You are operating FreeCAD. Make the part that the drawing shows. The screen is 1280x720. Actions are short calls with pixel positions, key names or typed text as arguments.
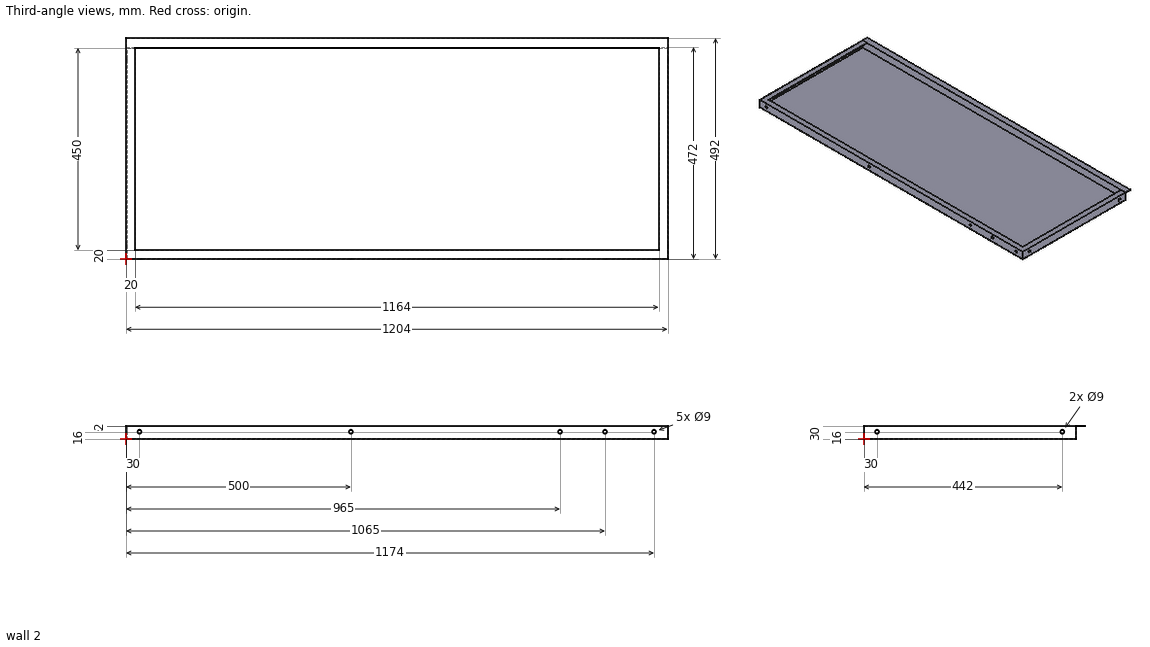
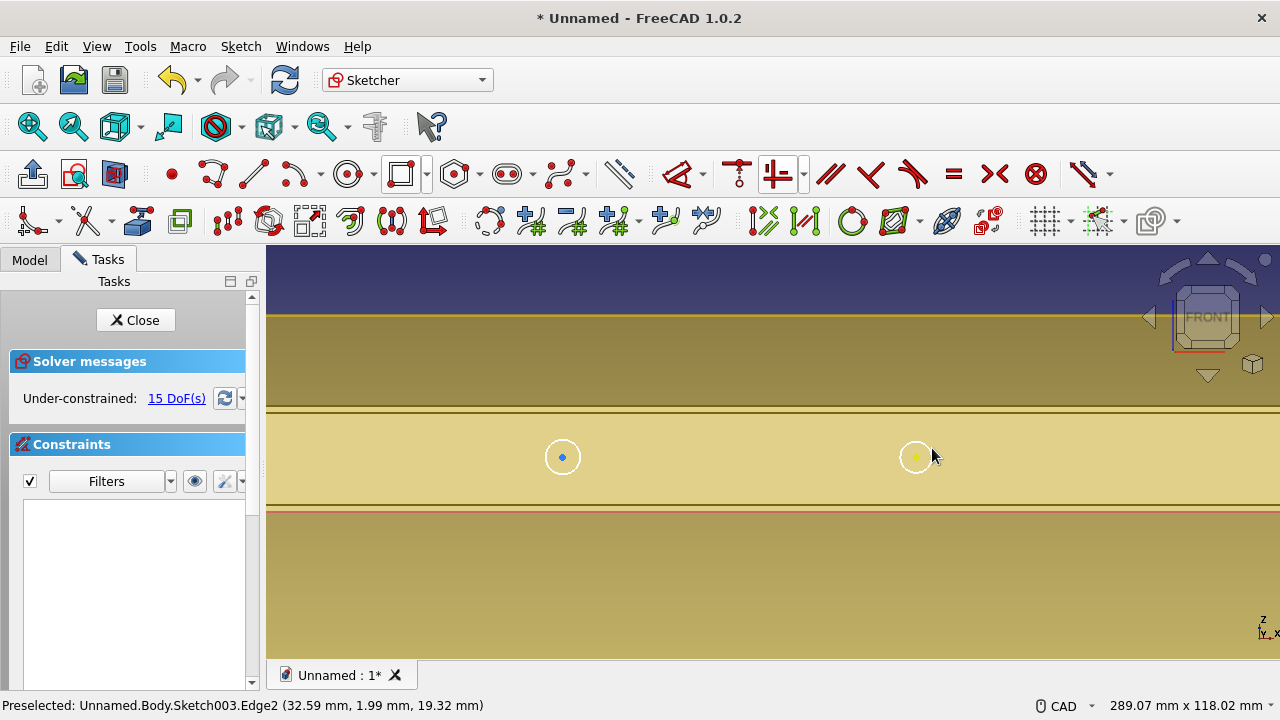
click(927, 446)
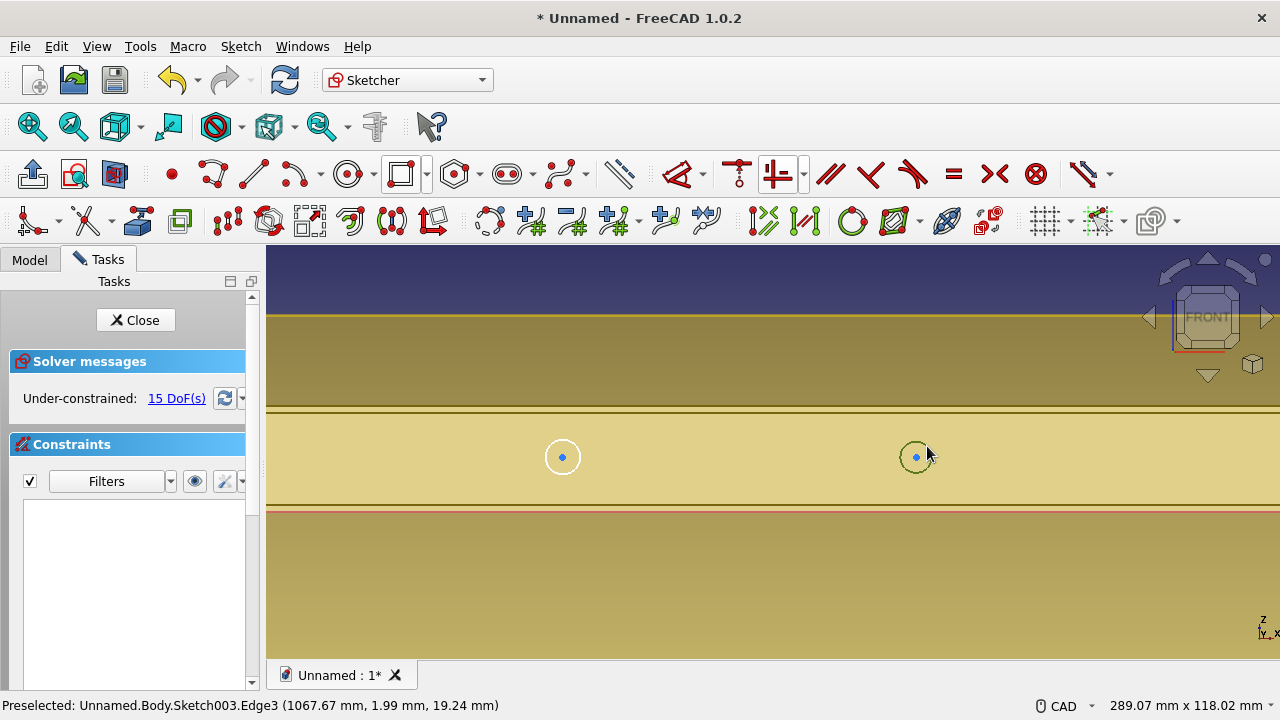
click(575, 445)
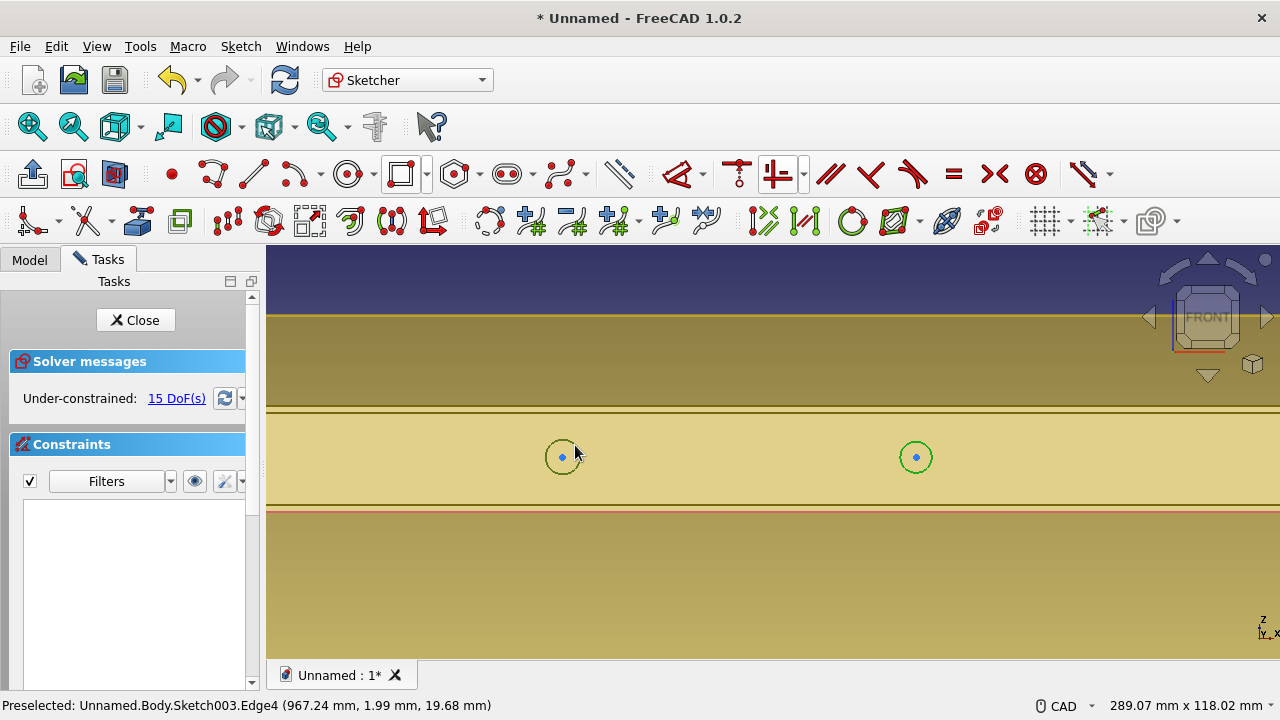
scroll(933, 448, down, 10)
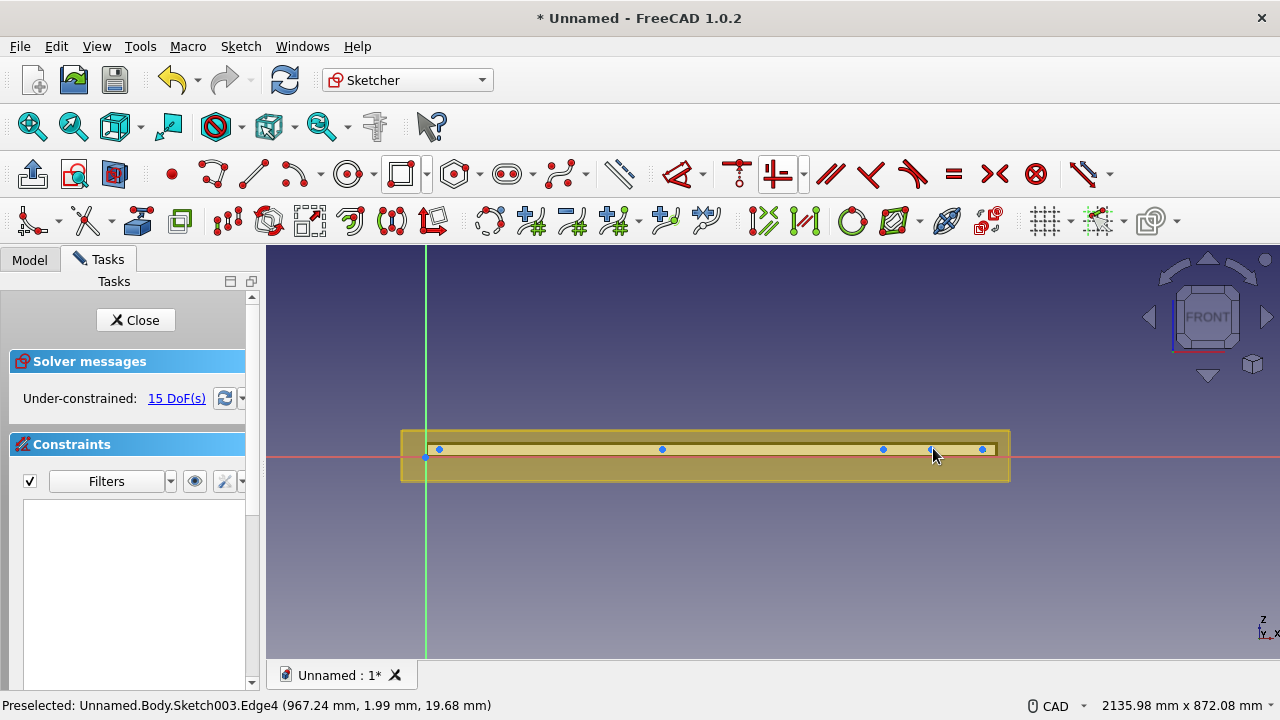
scroll(665, 448, up, 9)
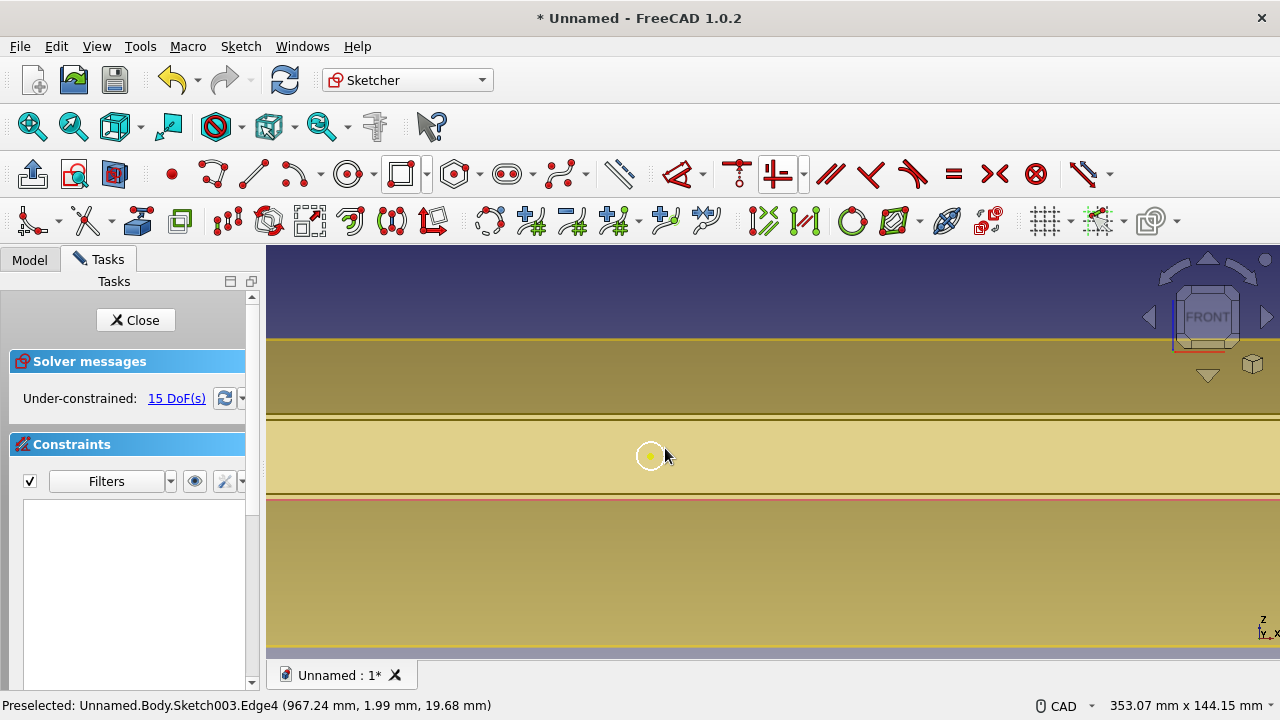
click(660, 446)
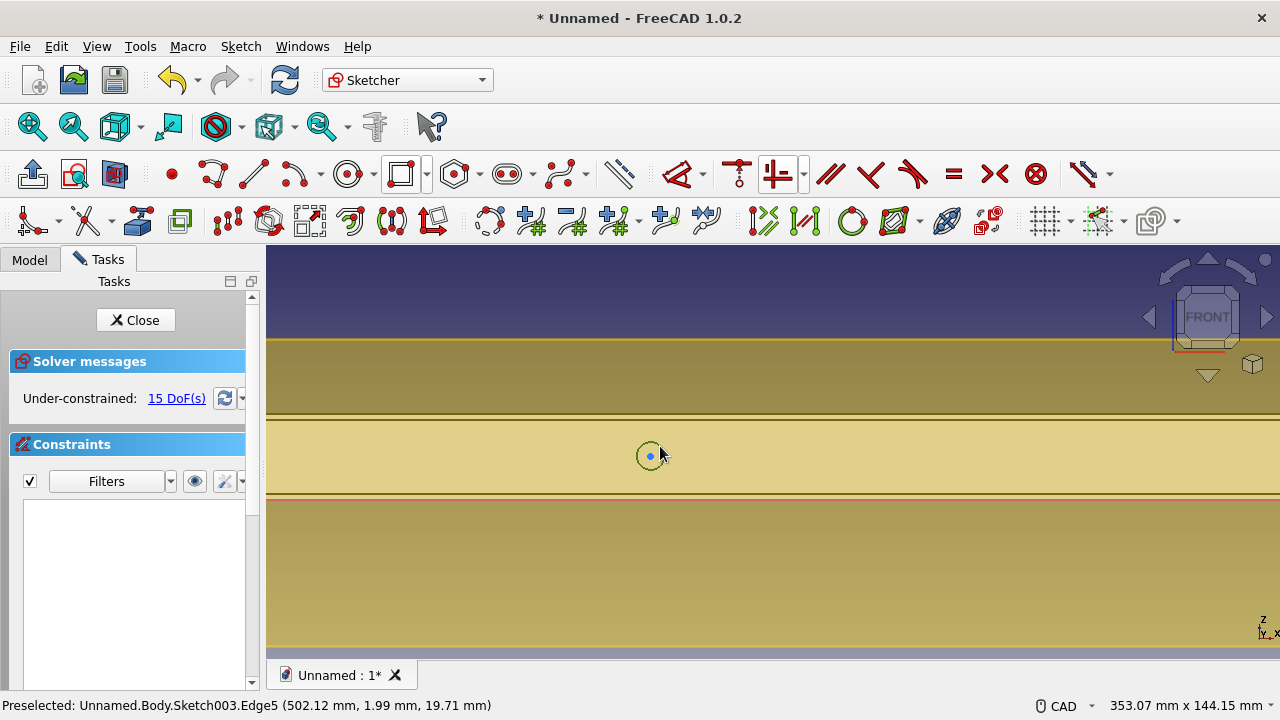
click(954, 174)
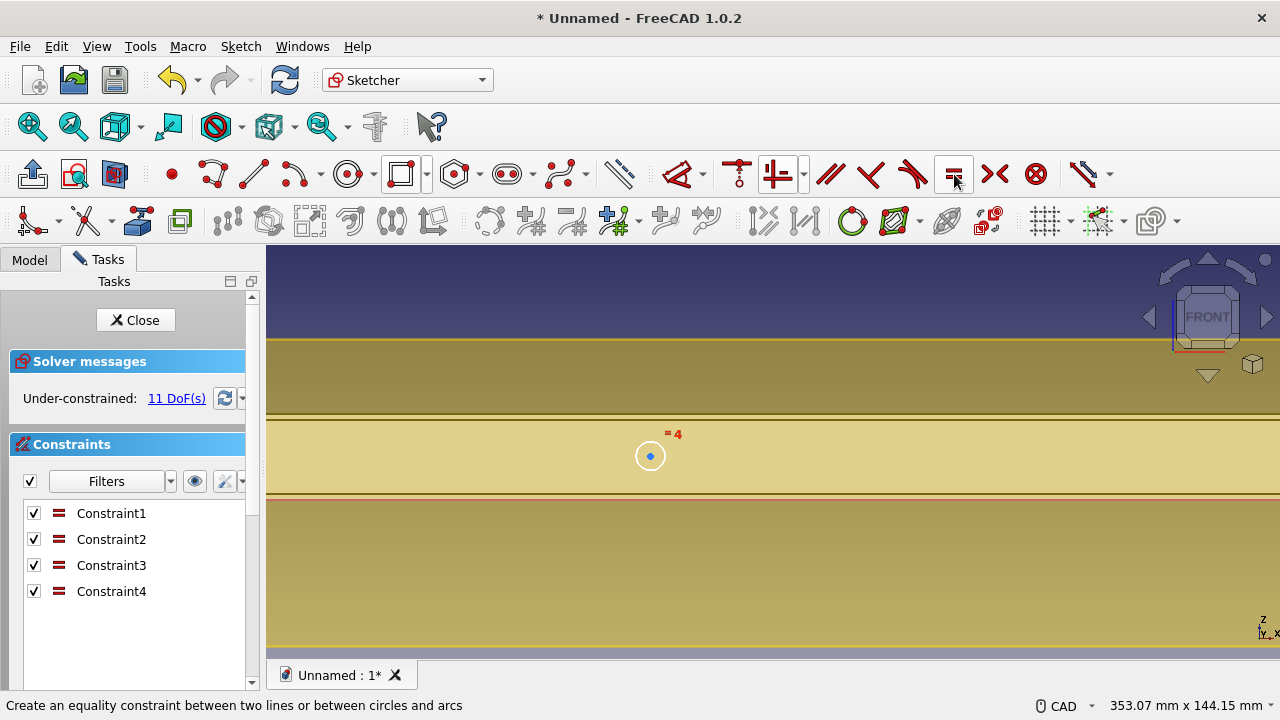
click(676, 174)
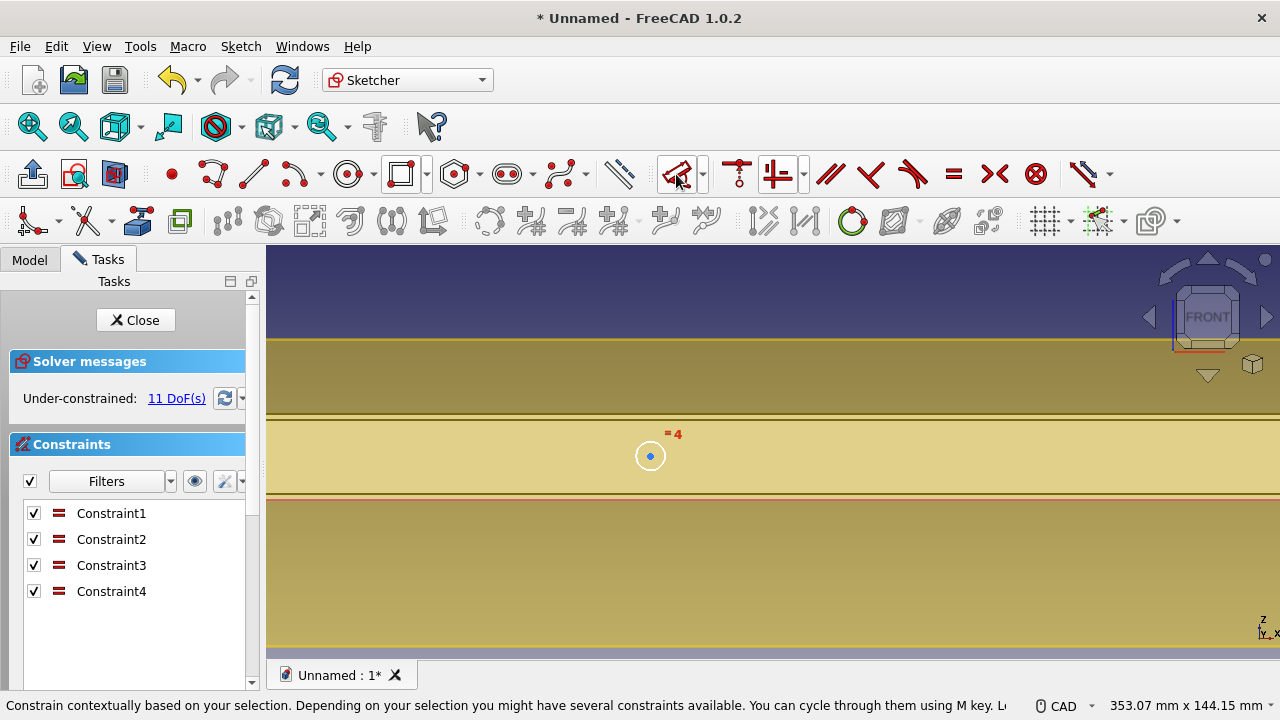
scroll(664, 448, down, 9)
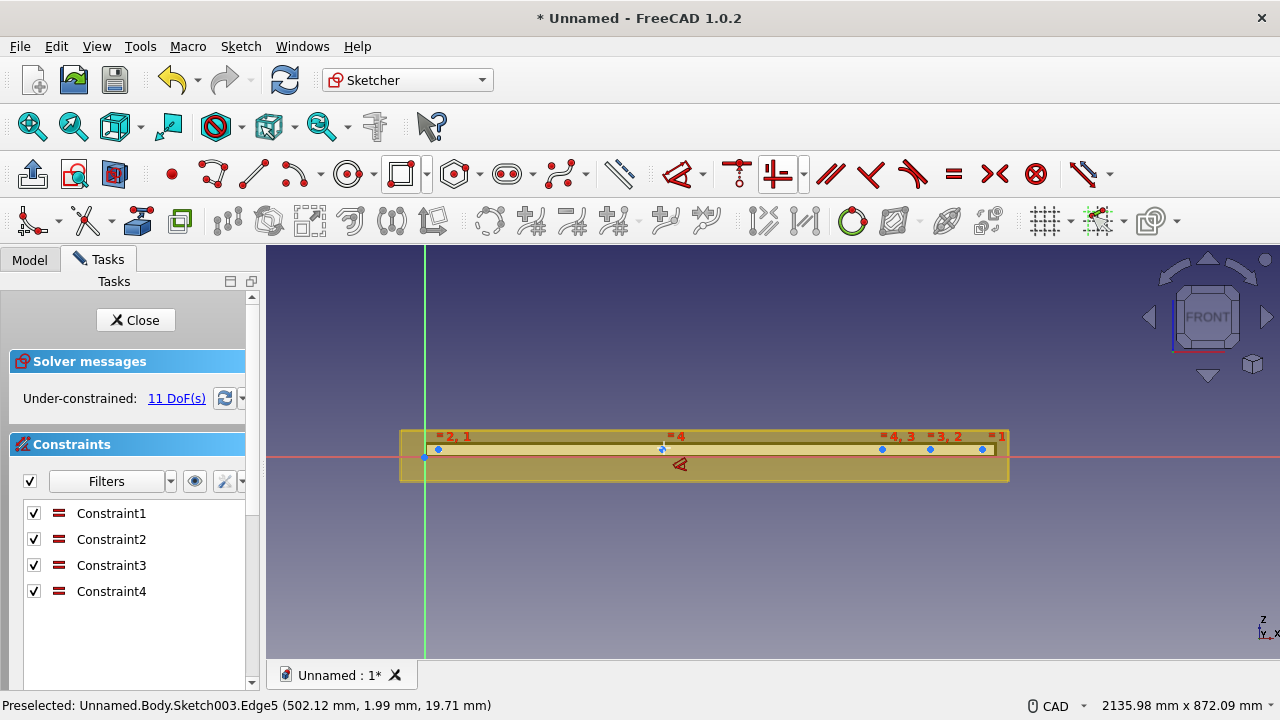
scroll(984, 448, up, 12)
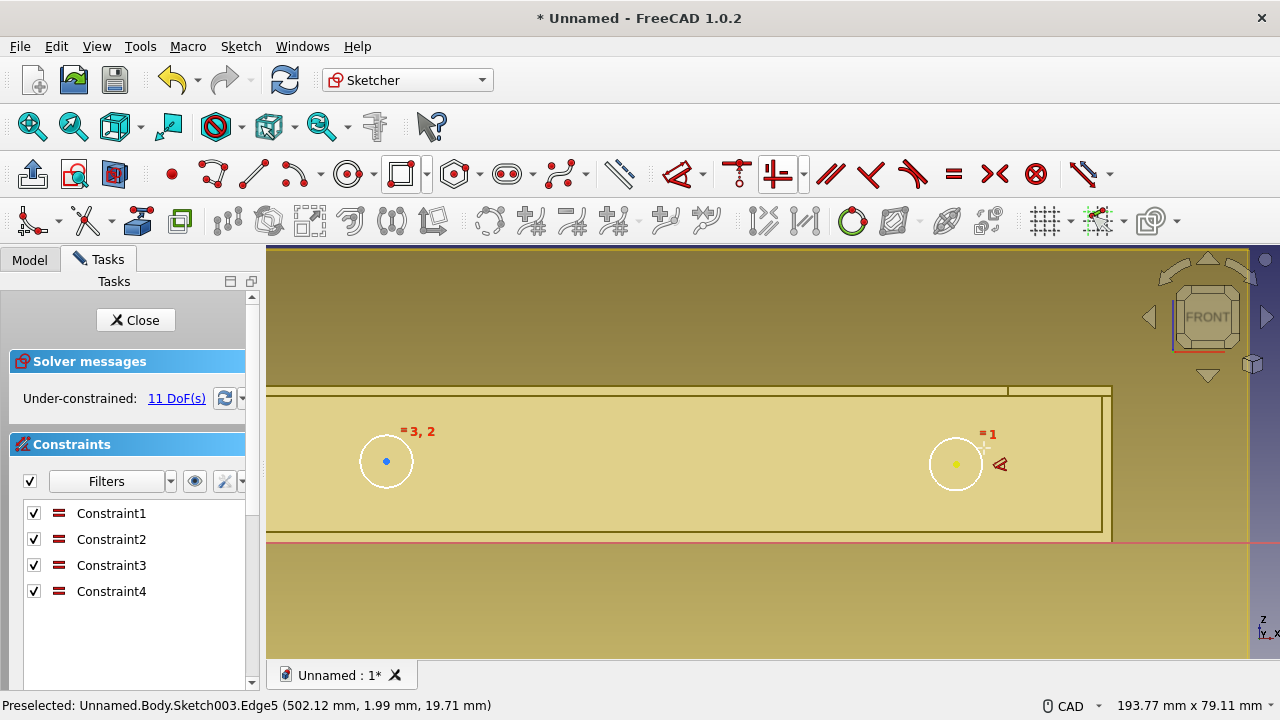
click(974, 446)
click(996, 423)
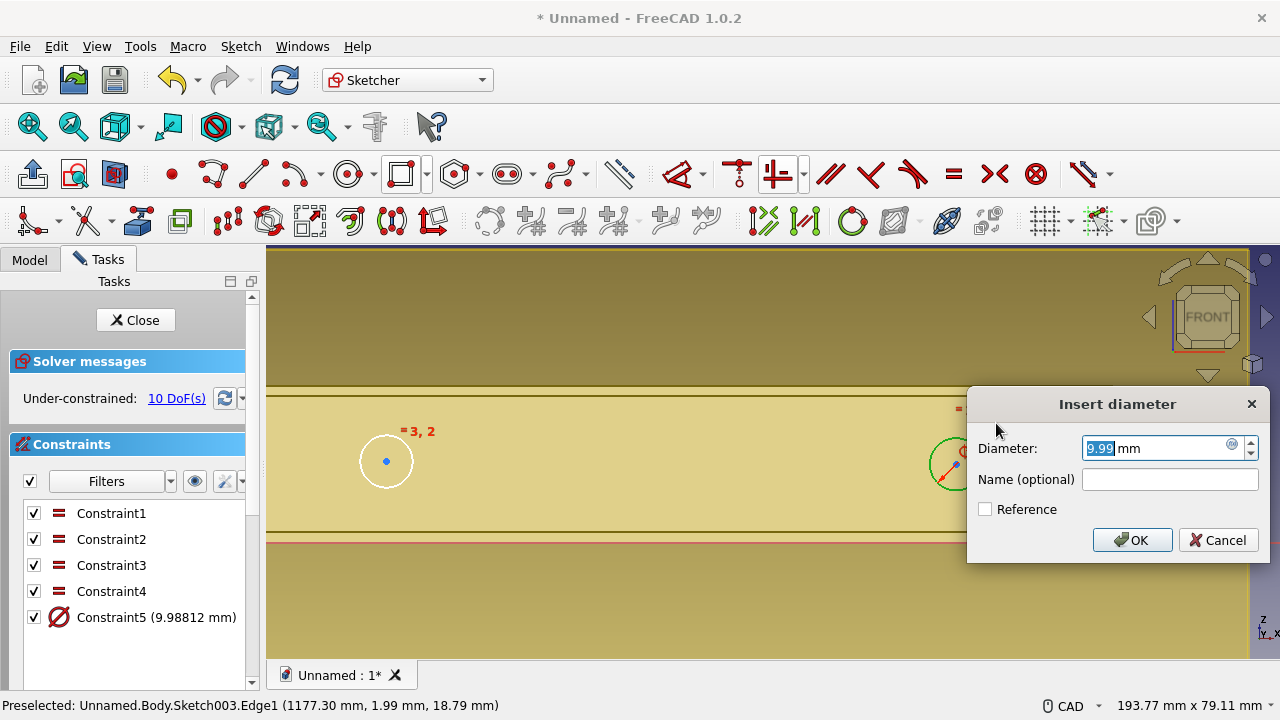
text(9)
key(Return)